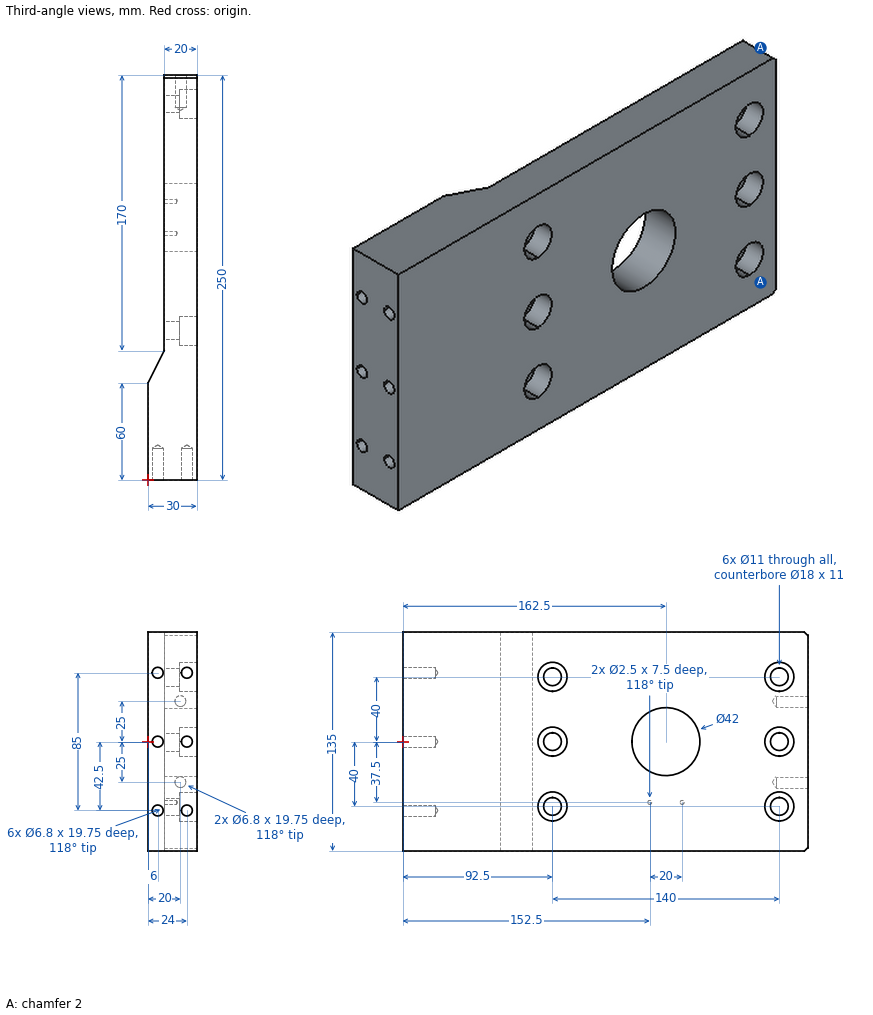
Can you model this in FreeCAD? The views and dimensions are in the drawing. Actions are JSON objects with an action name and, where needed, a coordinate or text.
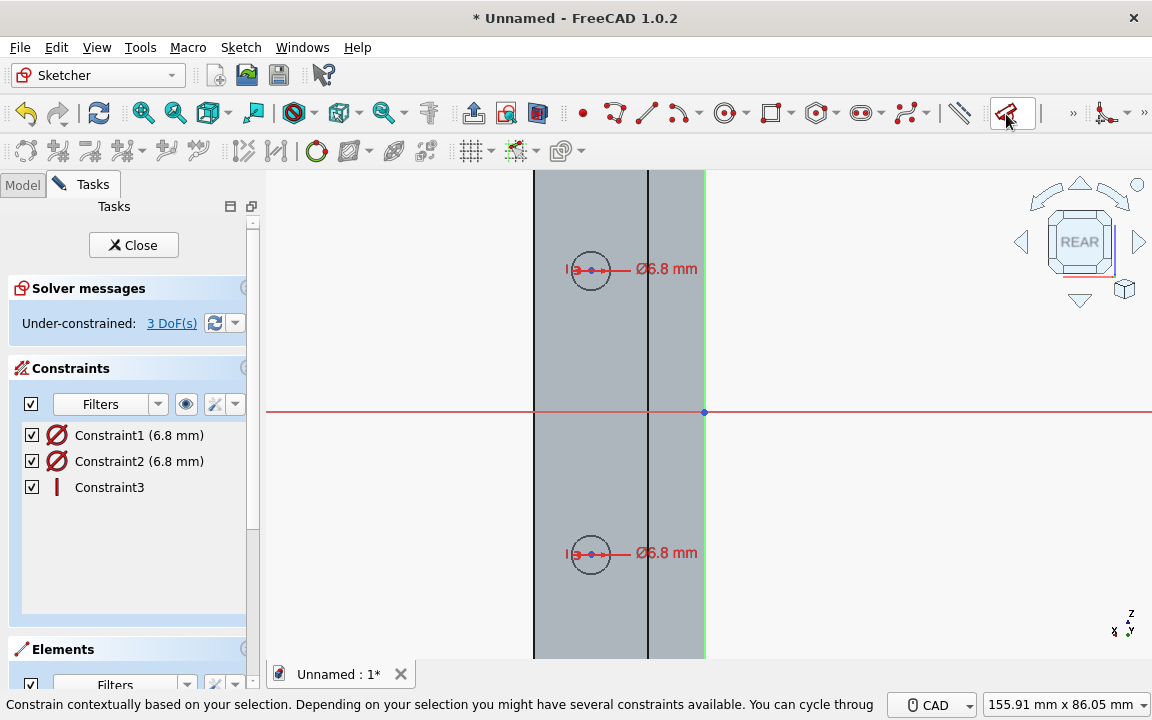
{"action": "left_click", "coordinate": [591, 555]}
{"action": "left_click", "coordinate": [648, 589]}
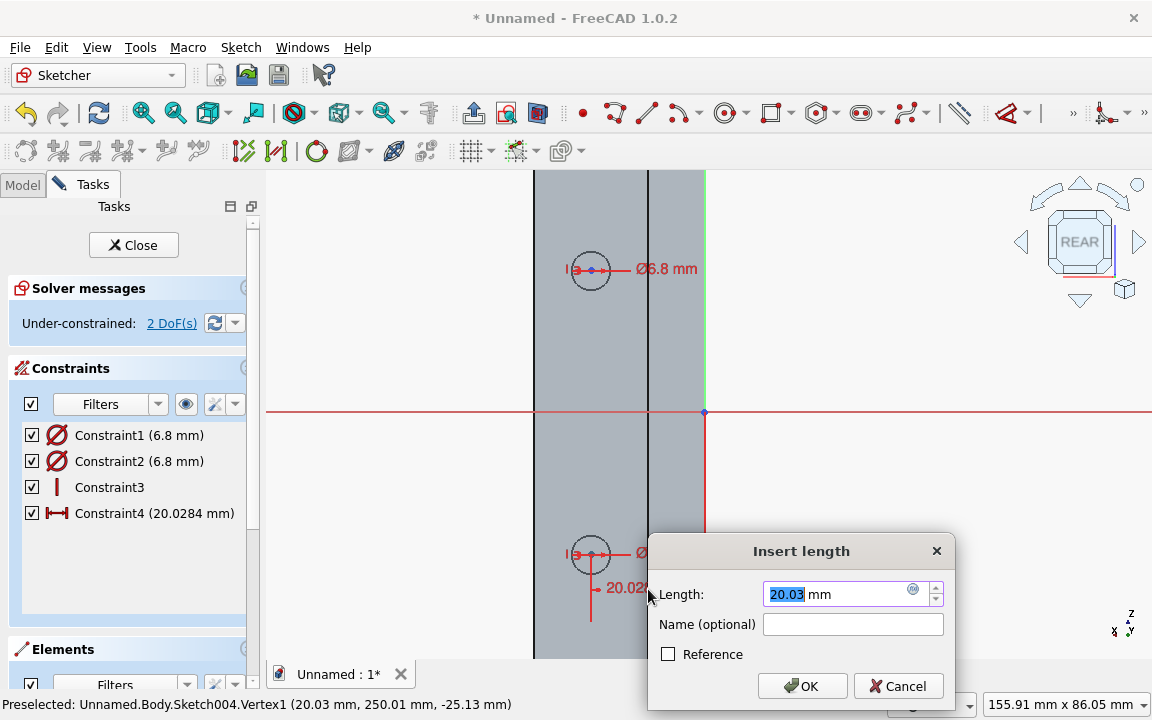
{"action": "type", "text": "20"}
{"action": "key", "text": "Return"}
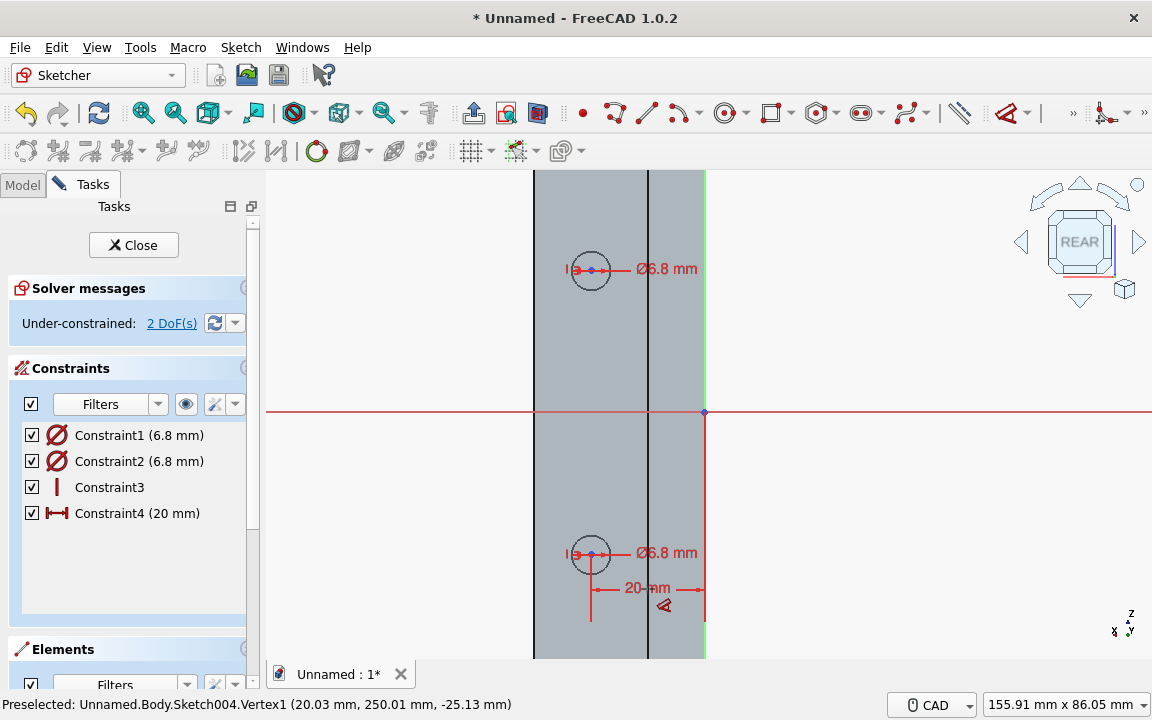
{"action": "left_click", "coordinate": [591, 555]}
{"action": "left_click", "coordinate": [739, 484]}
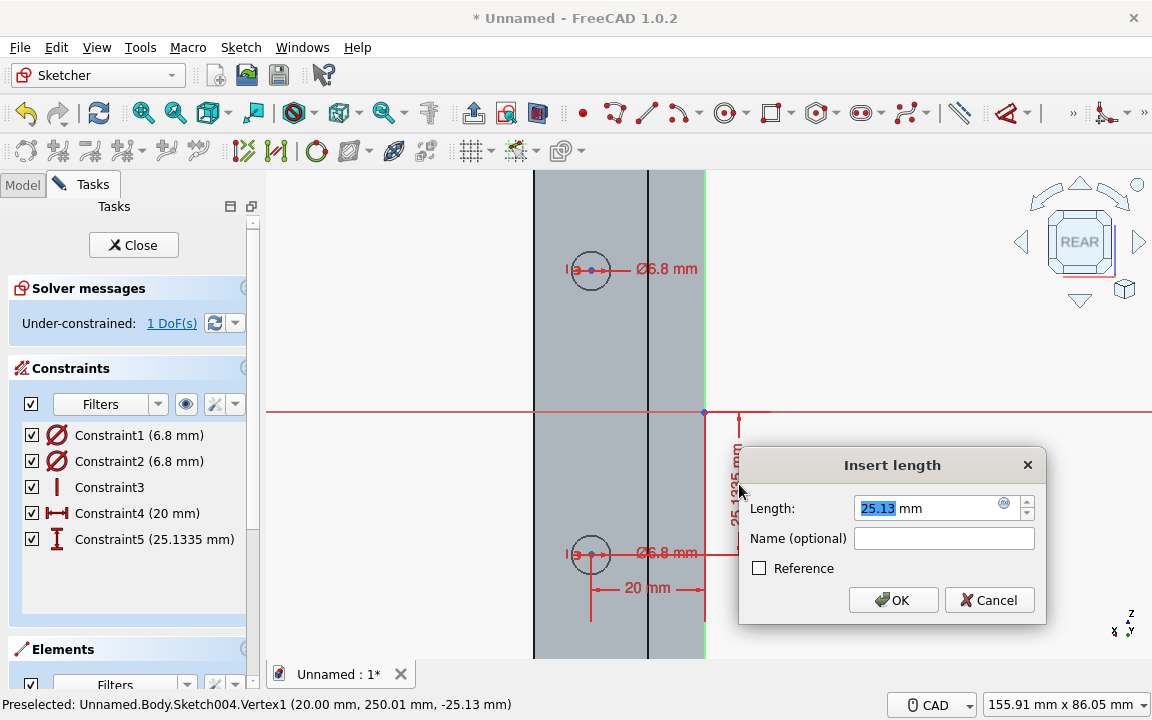
{"action": "type", "text": "25"}
{"action": "key", "text": "Return"}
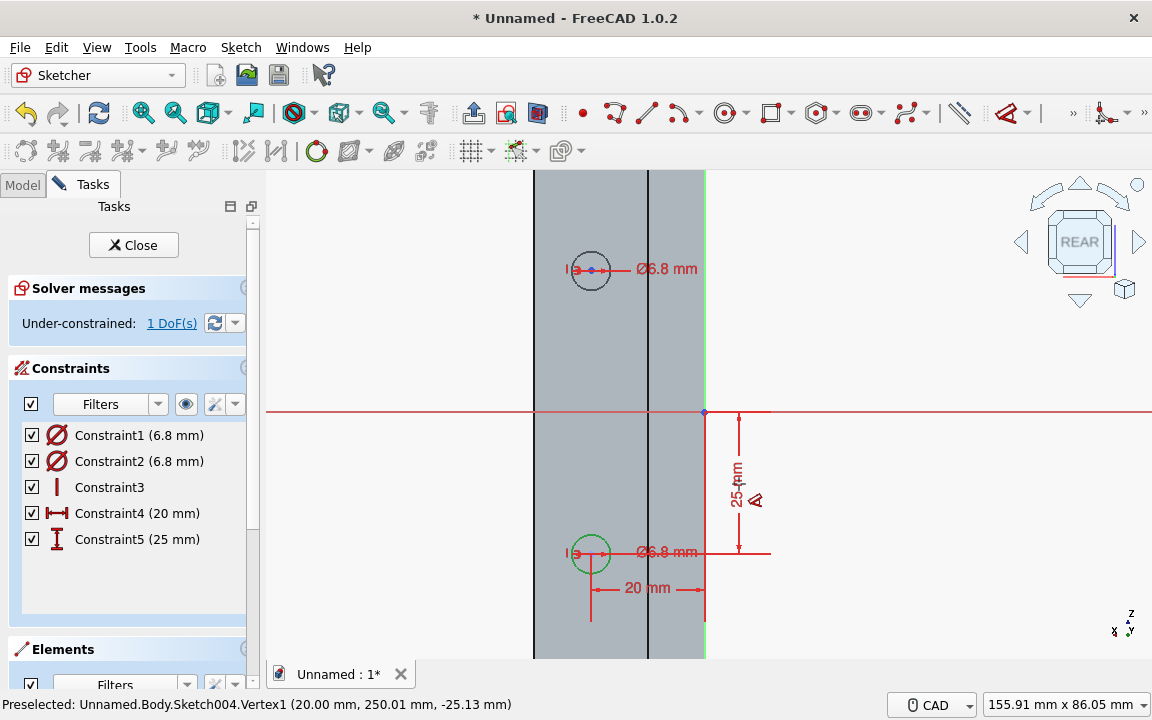
{"action": "left_click", "coordinate": [591, 271]}
{"action": "left_click", "coordinate": [739, 342]}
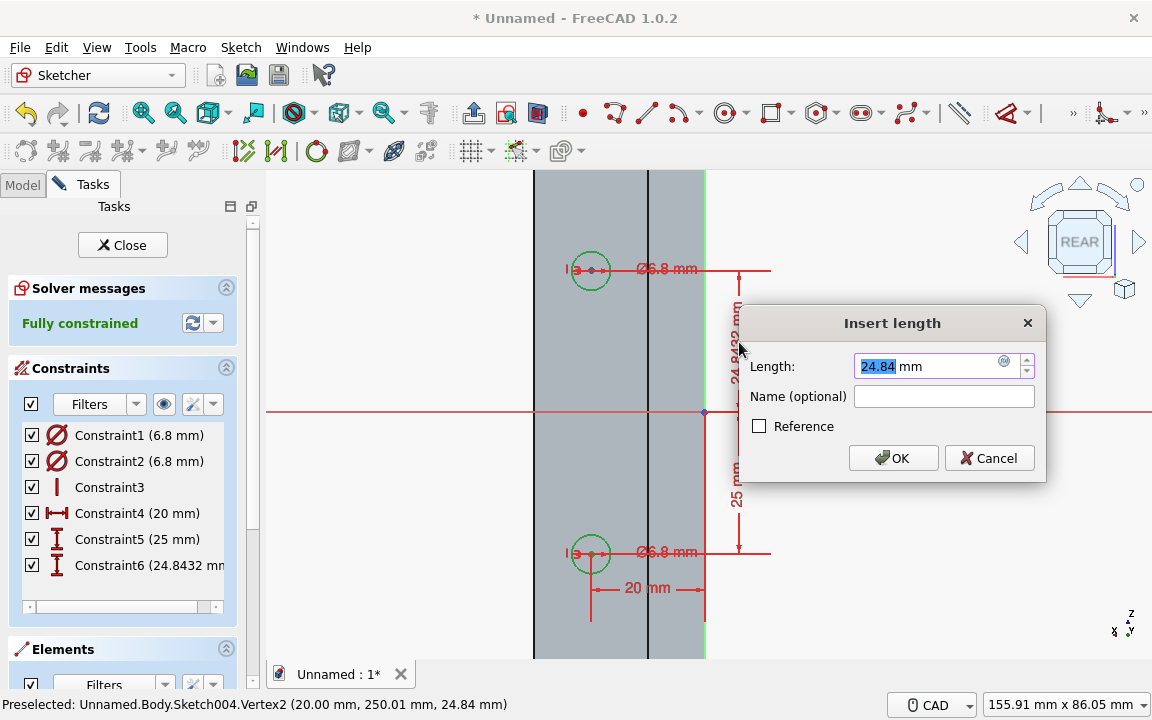
{"action": "type", "text": "25"}
{"action": "key", "text": "Return"}
{"action": "key", "text": "Escape"}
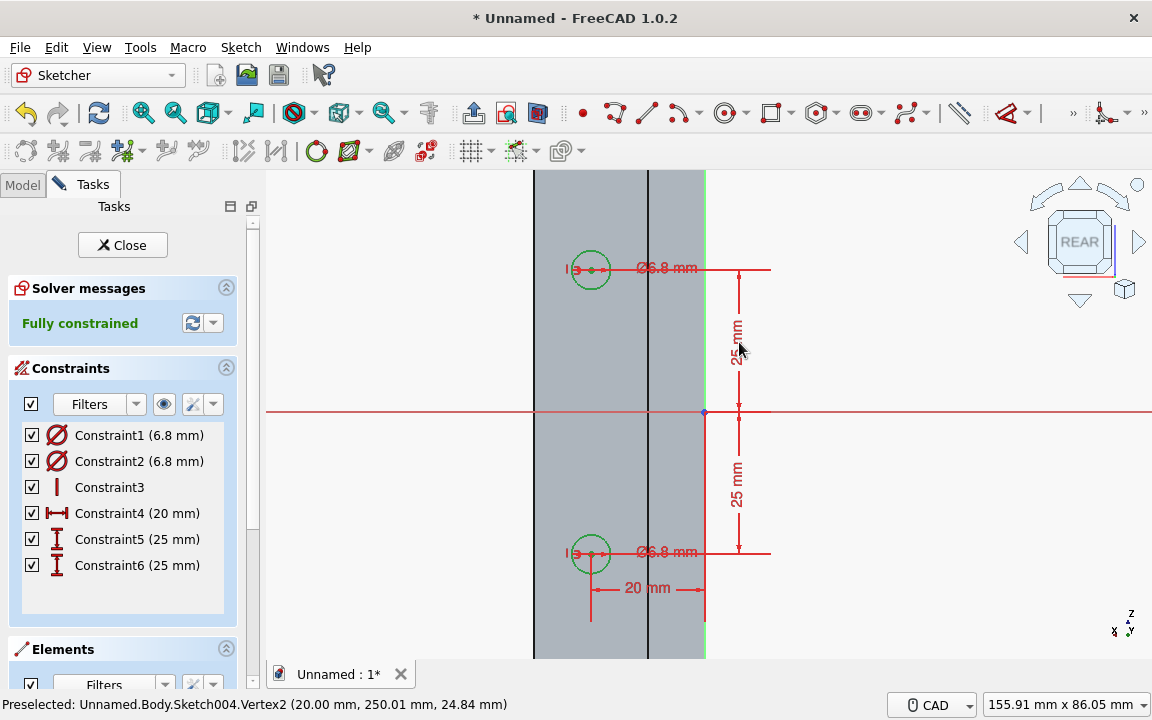
{"action": "left_click", "coordinate": [123, 245]}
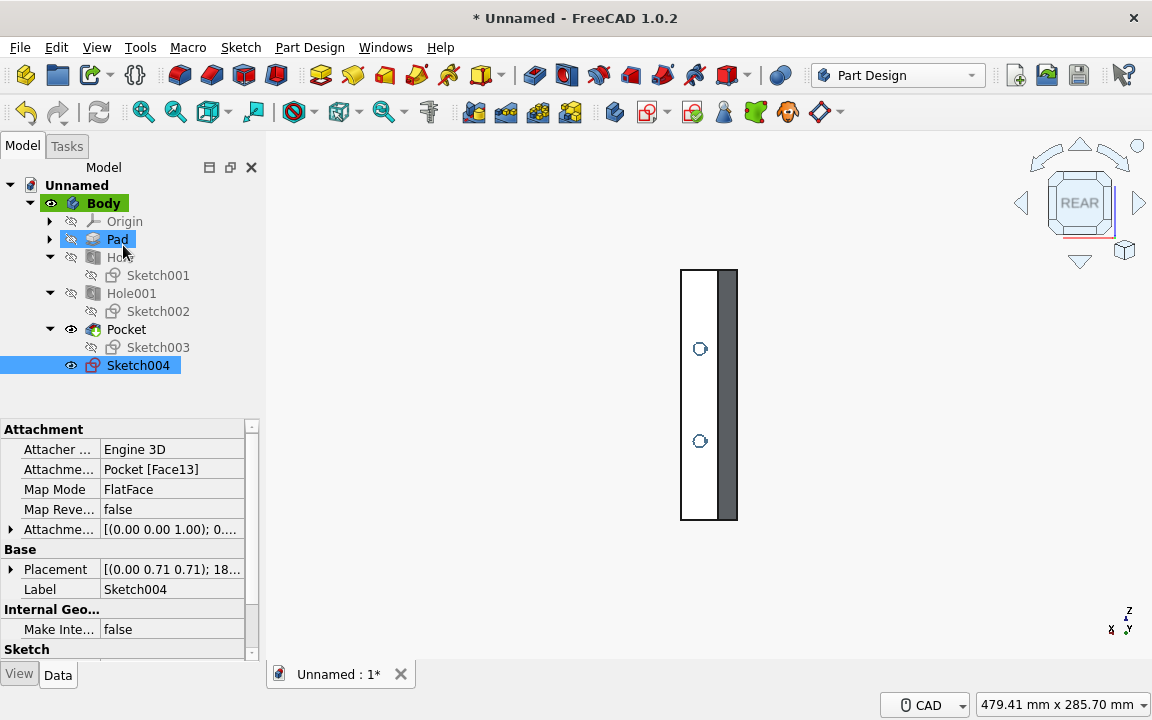
{"action": "left_click", "coordinate": [568, 76]}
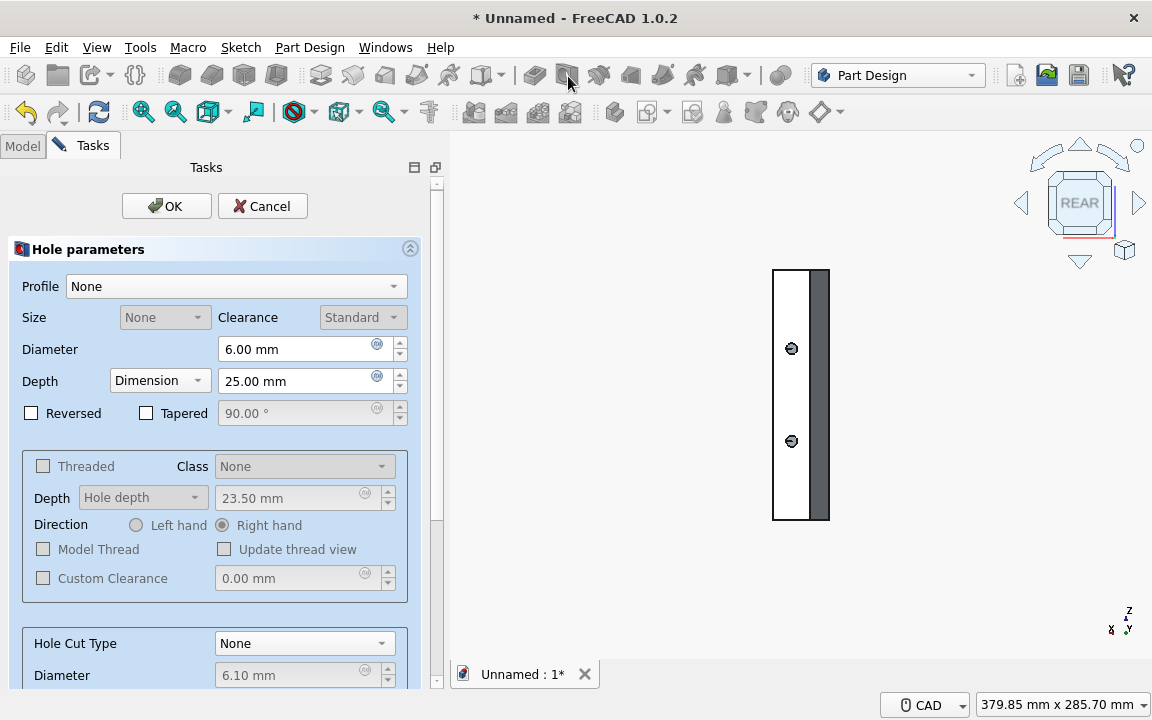
{"action": "triple_click", "coordinate": [305, 349]}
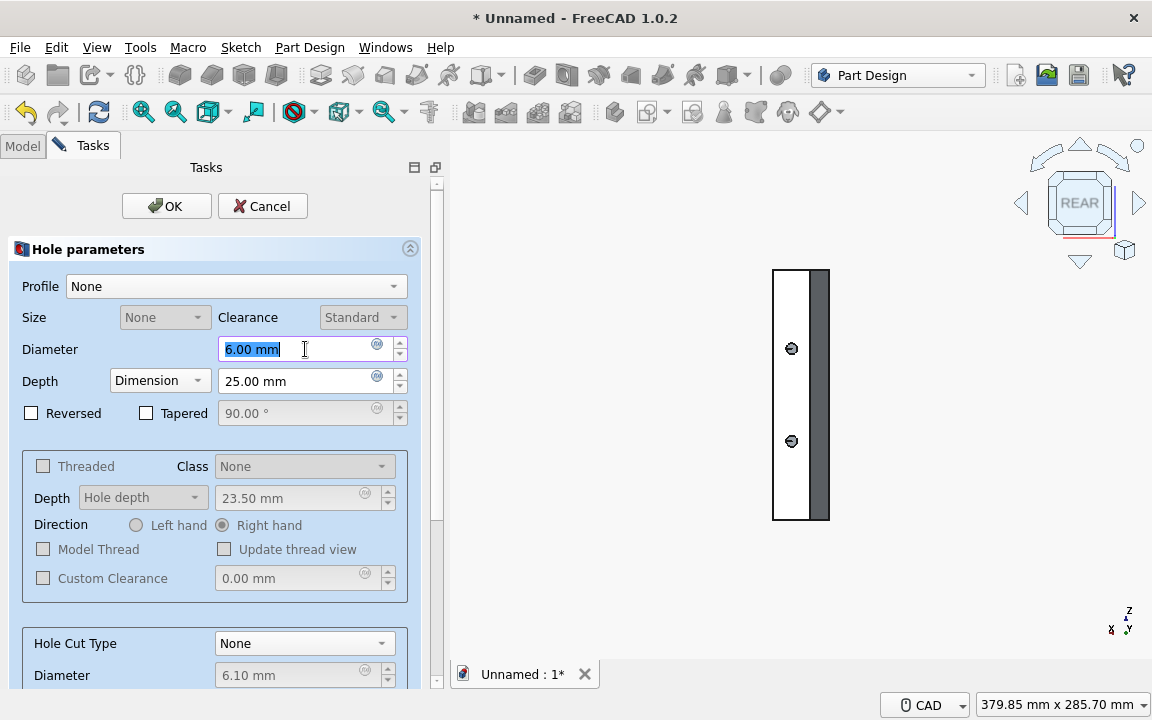
{"action": "type", "text": "6.8"}
{"action": "key", "text": "Tab"}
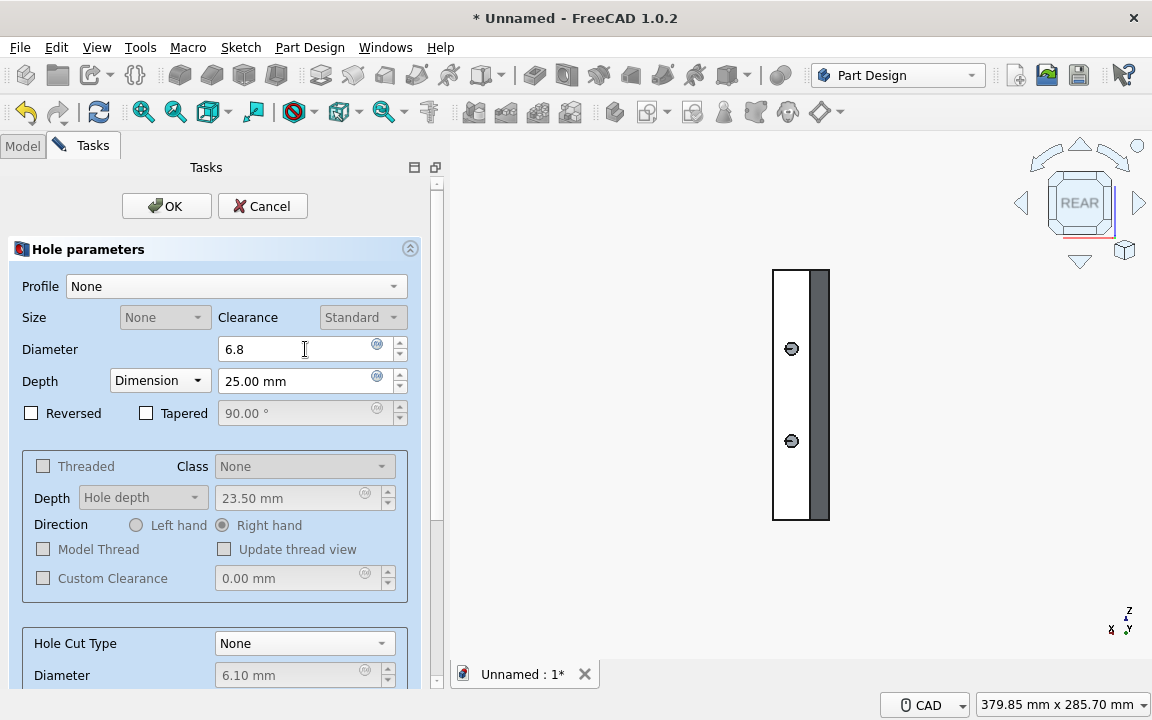
{"action": "triple_click", "coordinate": [305, 381]}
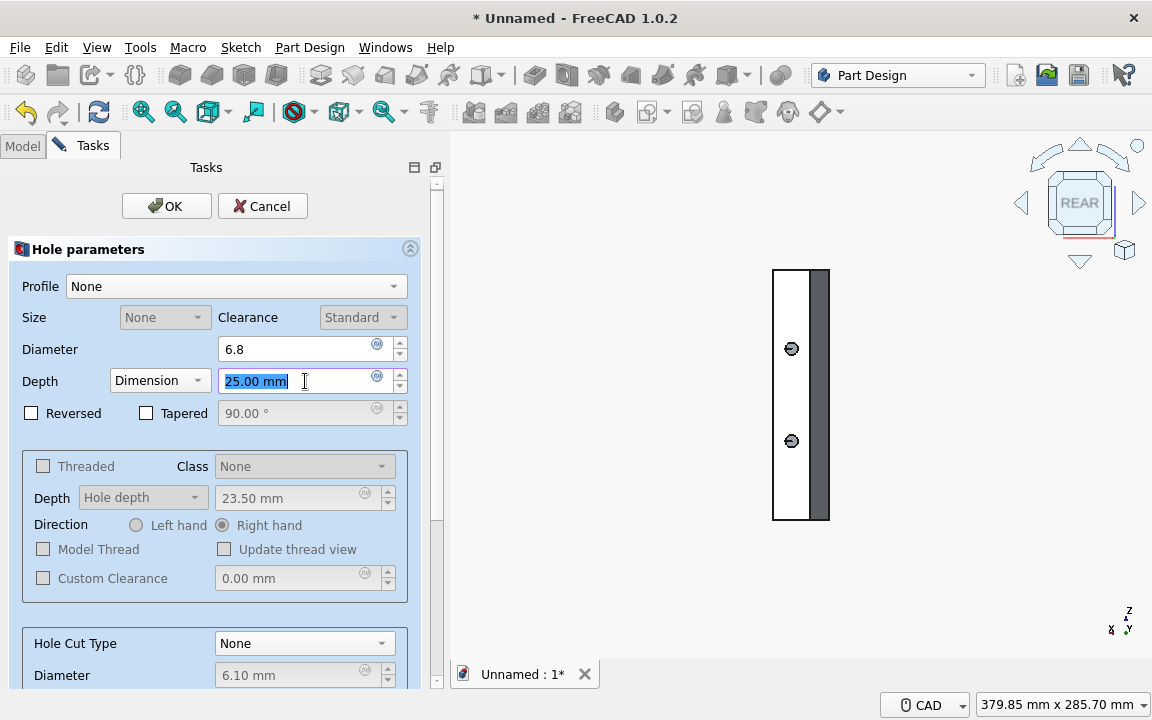
{"action": "type", "text": "19.75"}
{"action": "key", "text": "Tab"}